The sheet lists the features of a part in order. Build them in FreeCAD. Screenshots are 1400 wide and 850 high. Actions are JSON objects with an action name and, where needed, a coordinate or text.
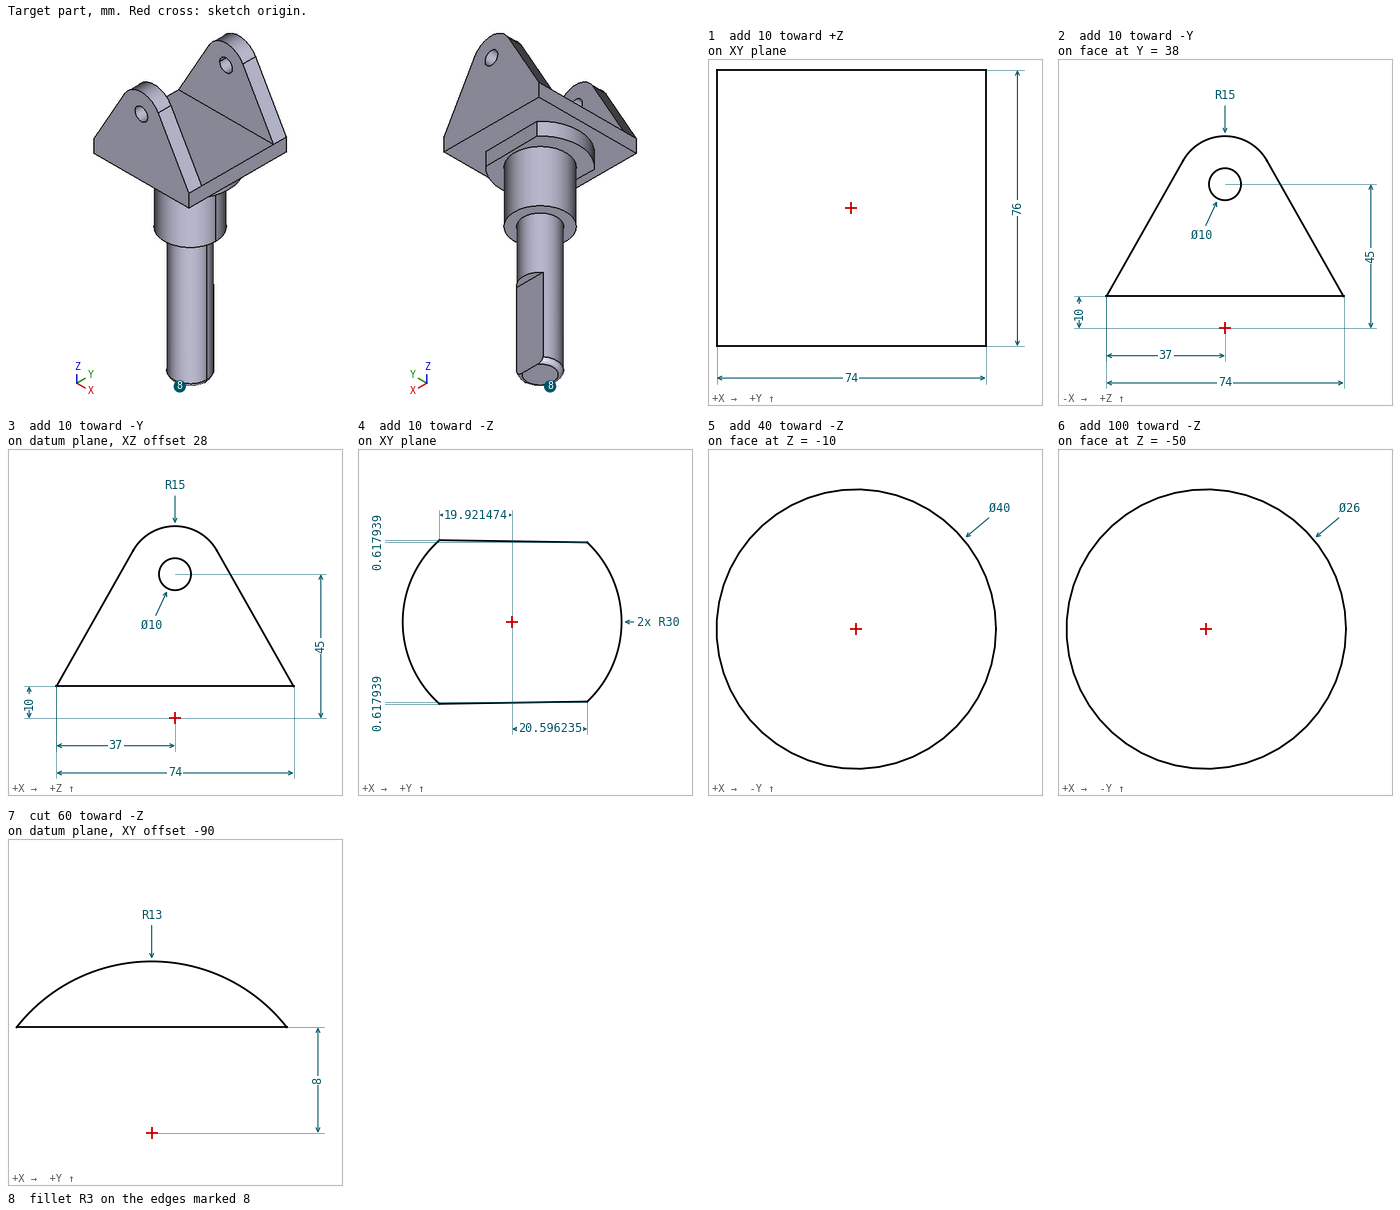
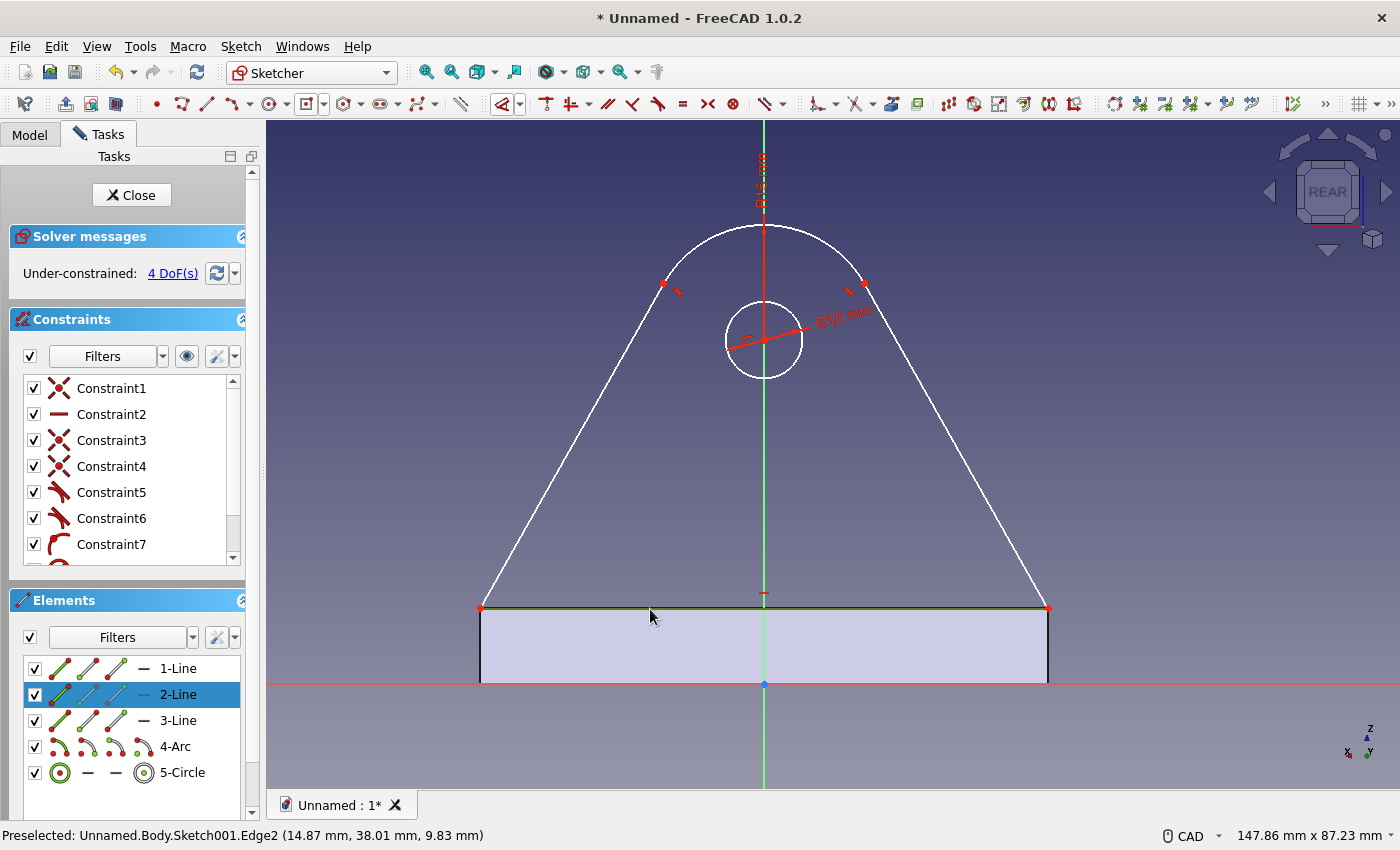
{"action": "left_click", "coordinate": [520, 104]}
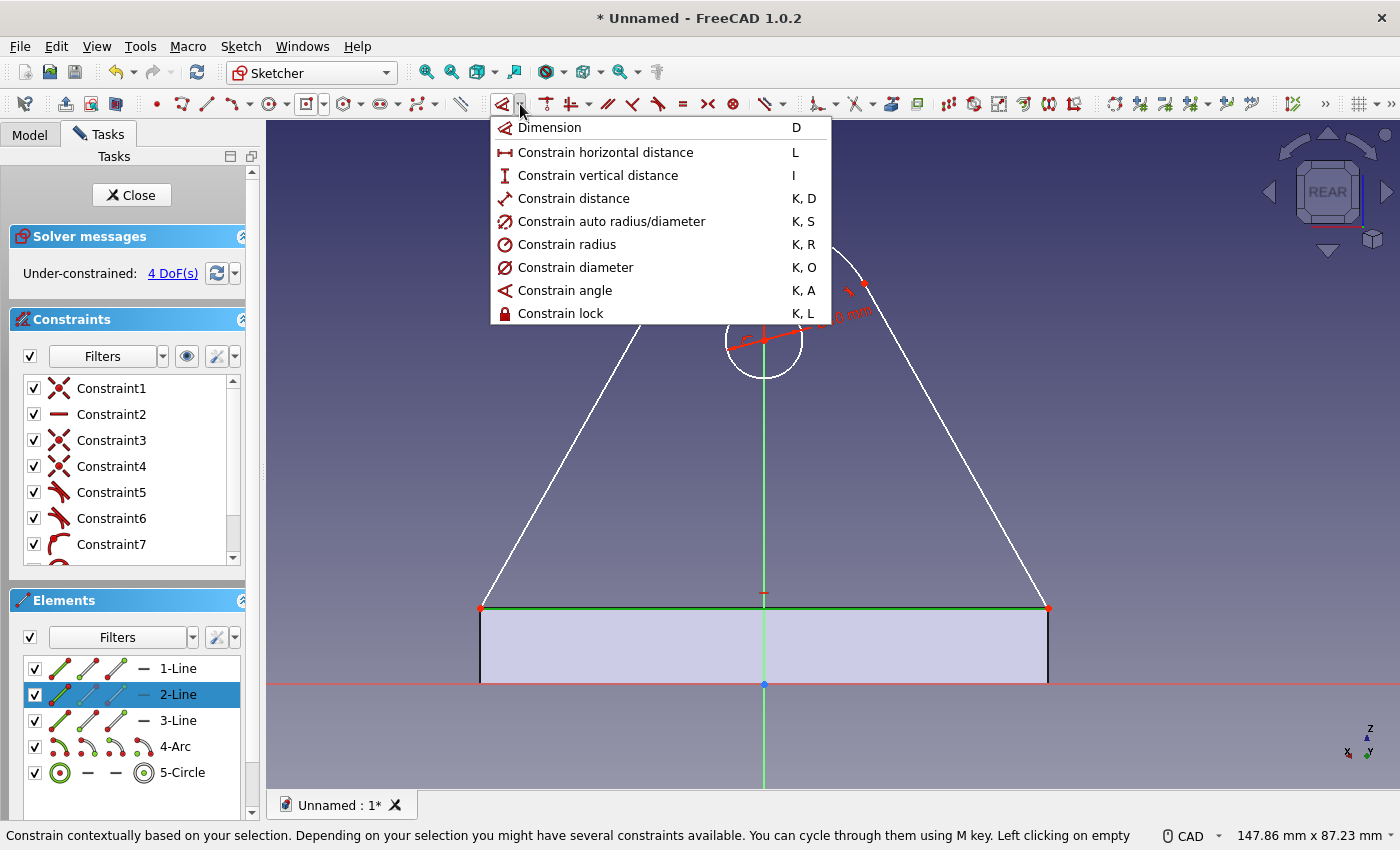
{"action": "left_click", "coordinate": [661, 152]}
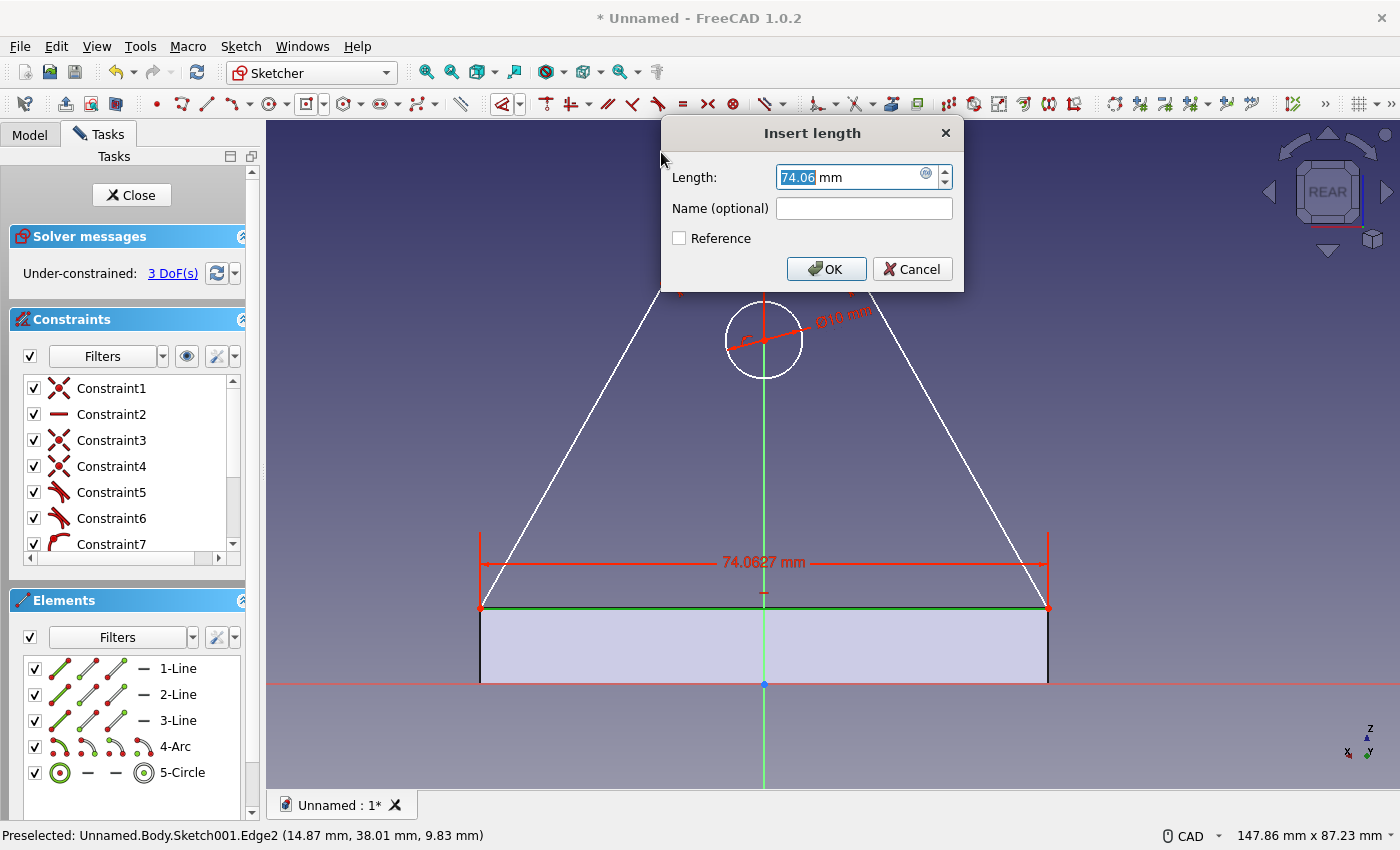
{"action": "type", "text": "74"}
{"action": "key", "text": "Return"}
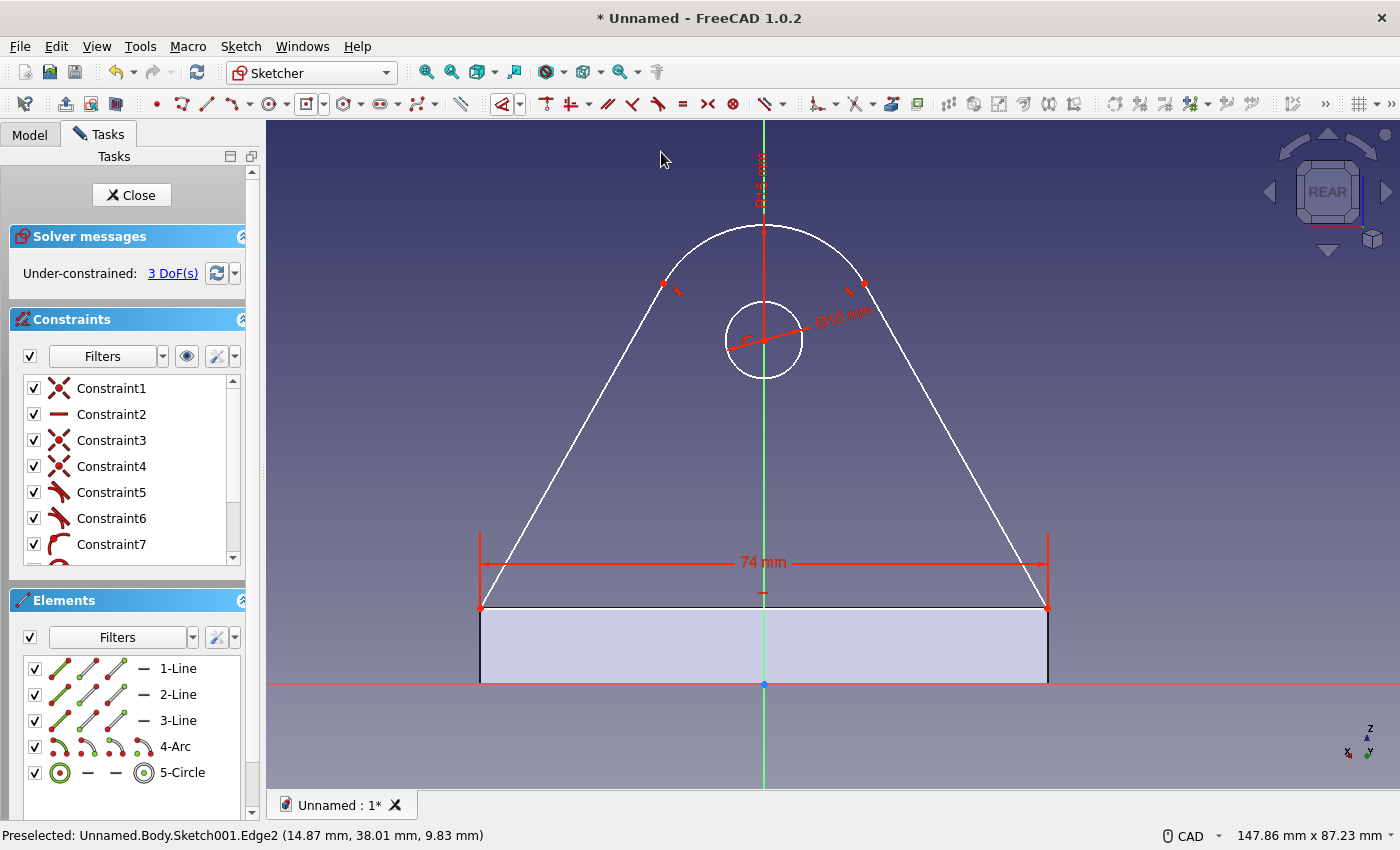
{"action": "left_click", "coordinate": [764, 340]}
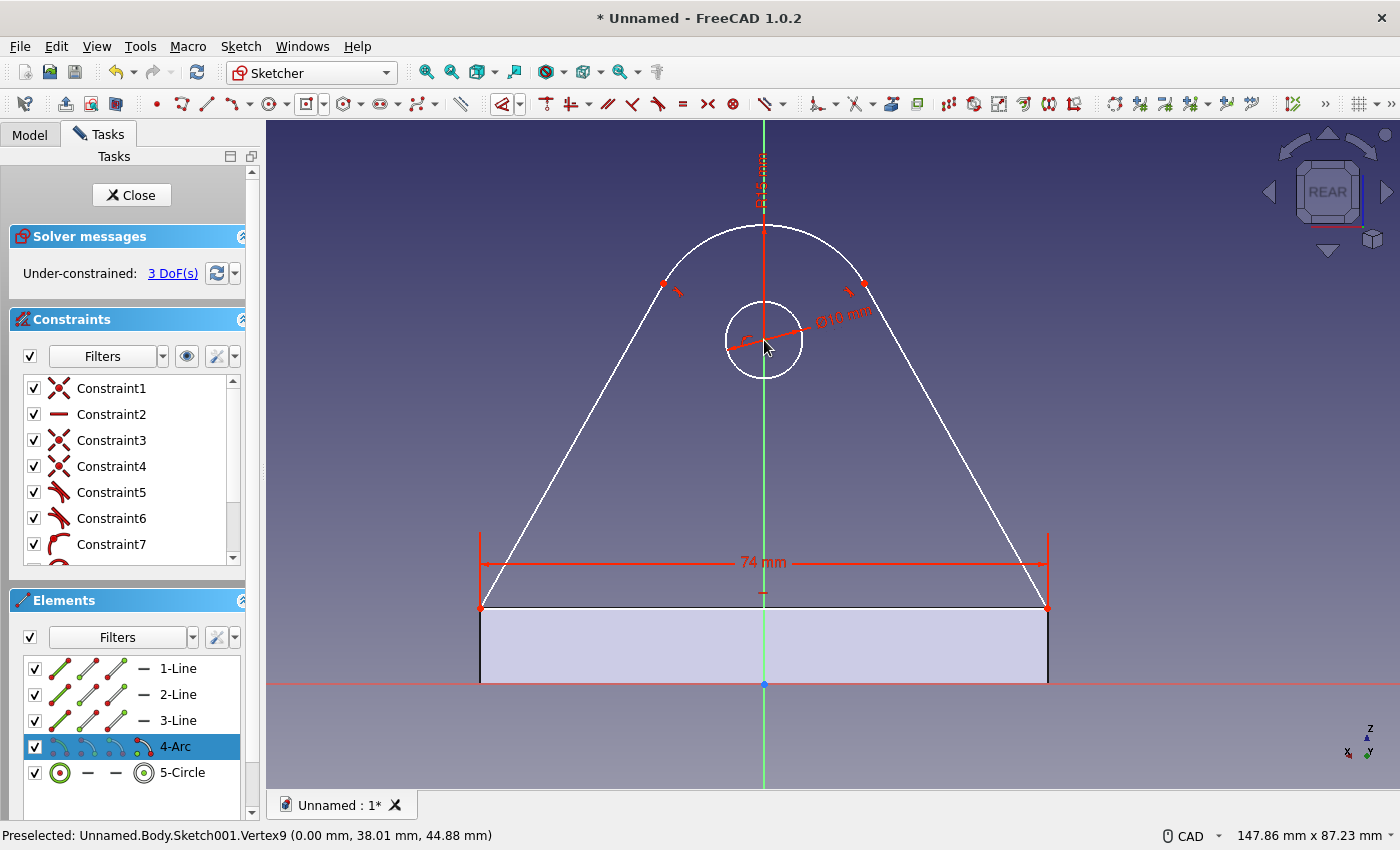
{"action": "key", "text": "i"}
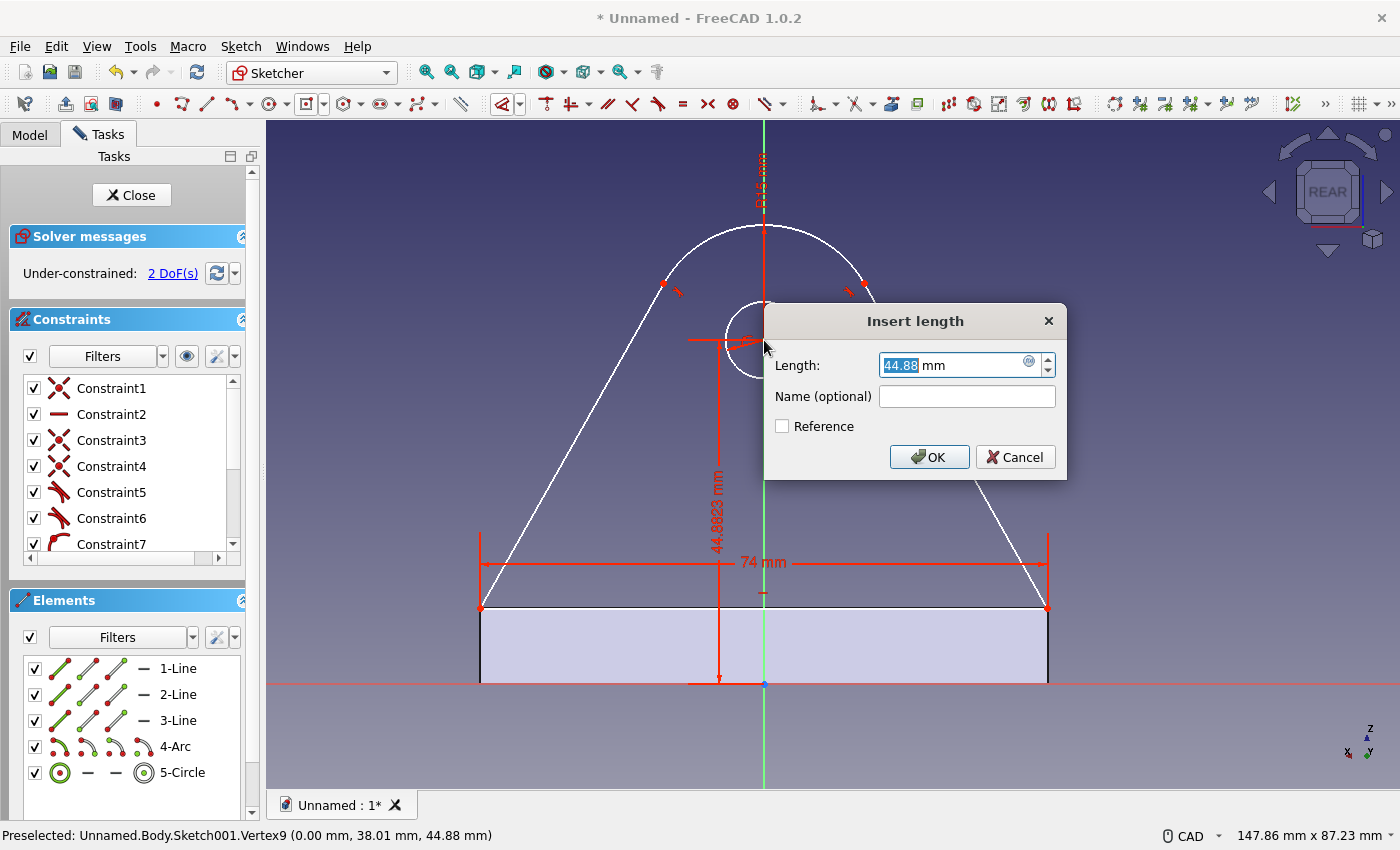
{"action": "type", "text": "45"}
{"action": "key", "text": "Return"}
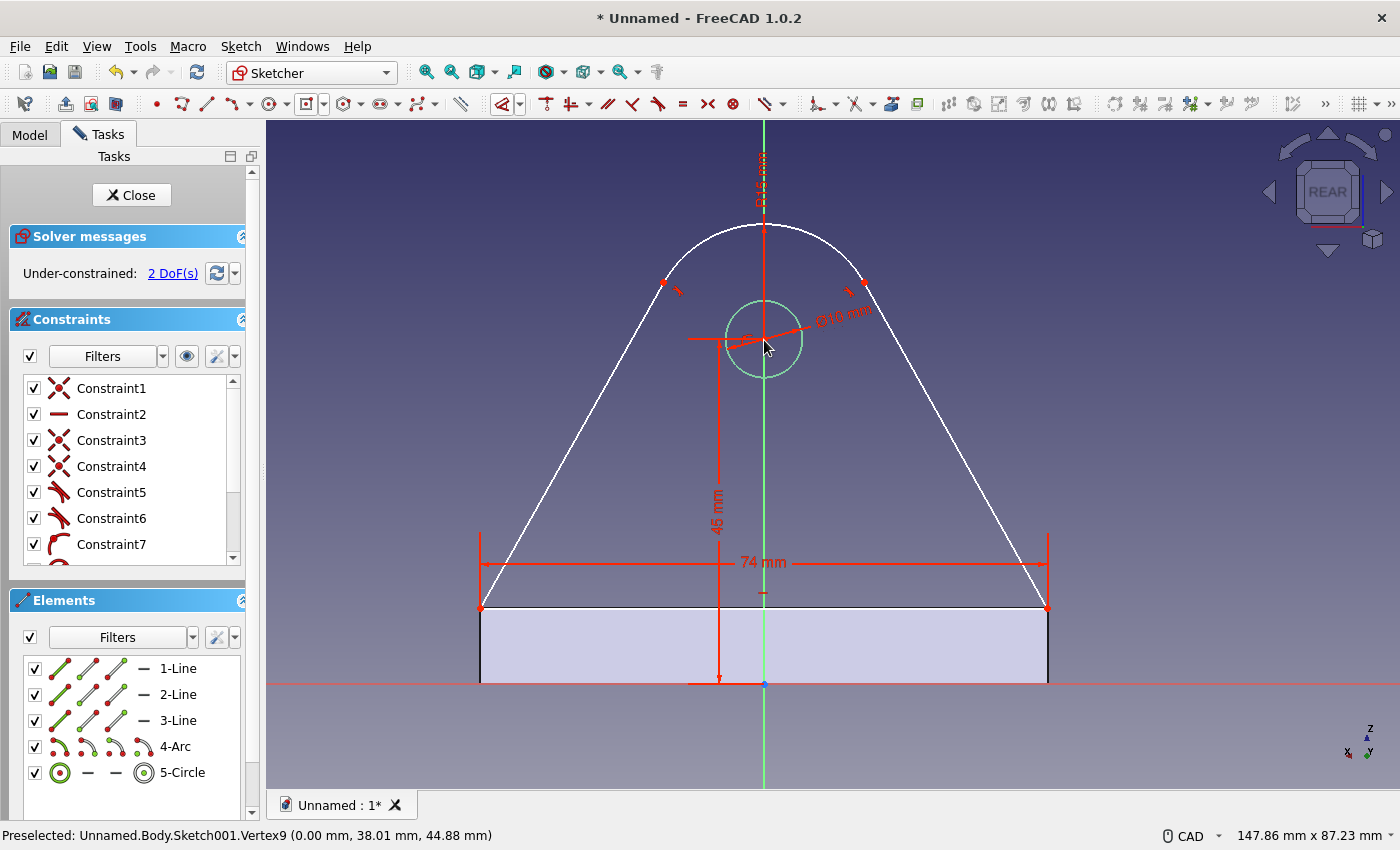
{"action": "left_click", "coordinate": [480, 609]}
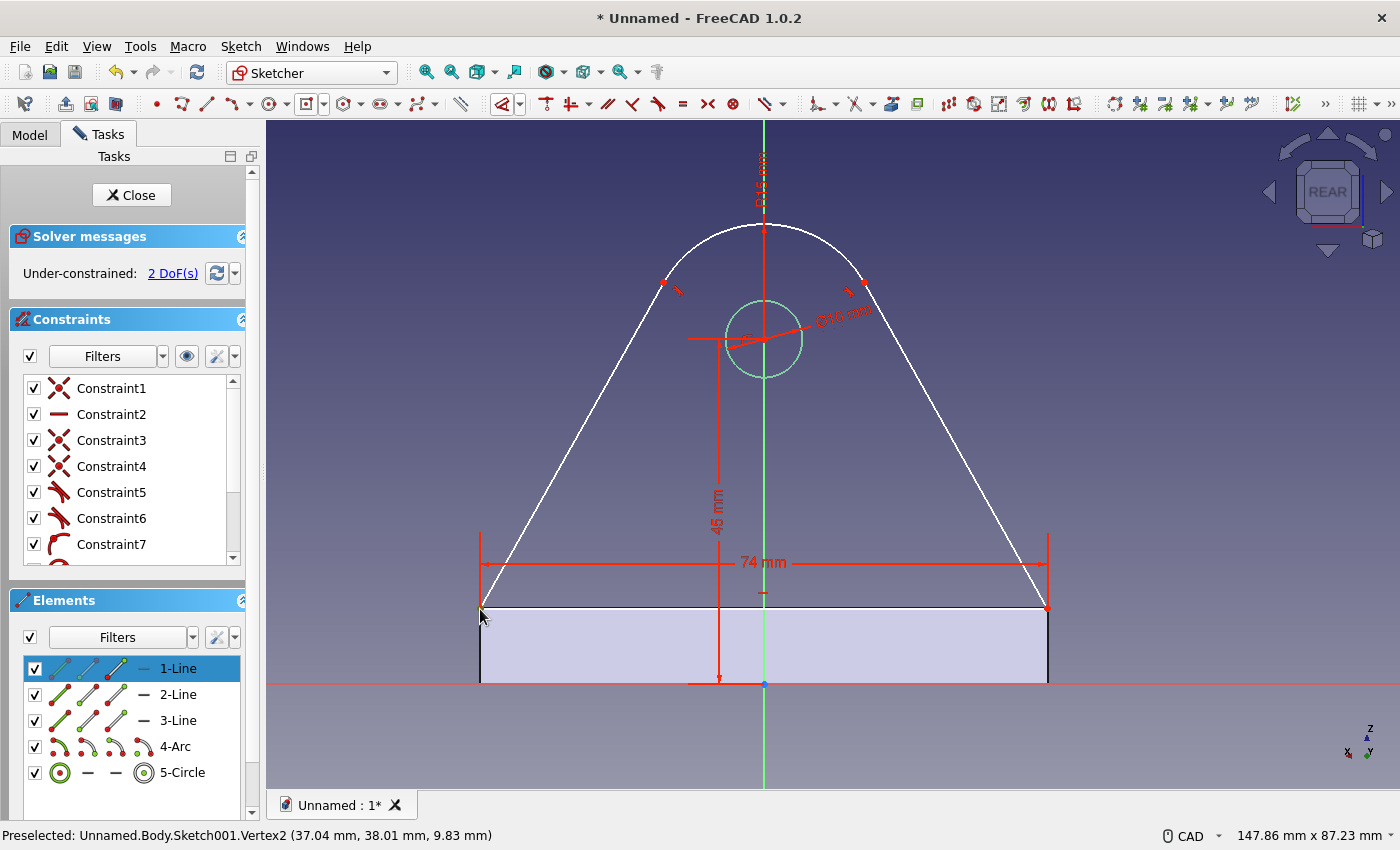
{"action": "left_click", "coordinate": [520, 104]}